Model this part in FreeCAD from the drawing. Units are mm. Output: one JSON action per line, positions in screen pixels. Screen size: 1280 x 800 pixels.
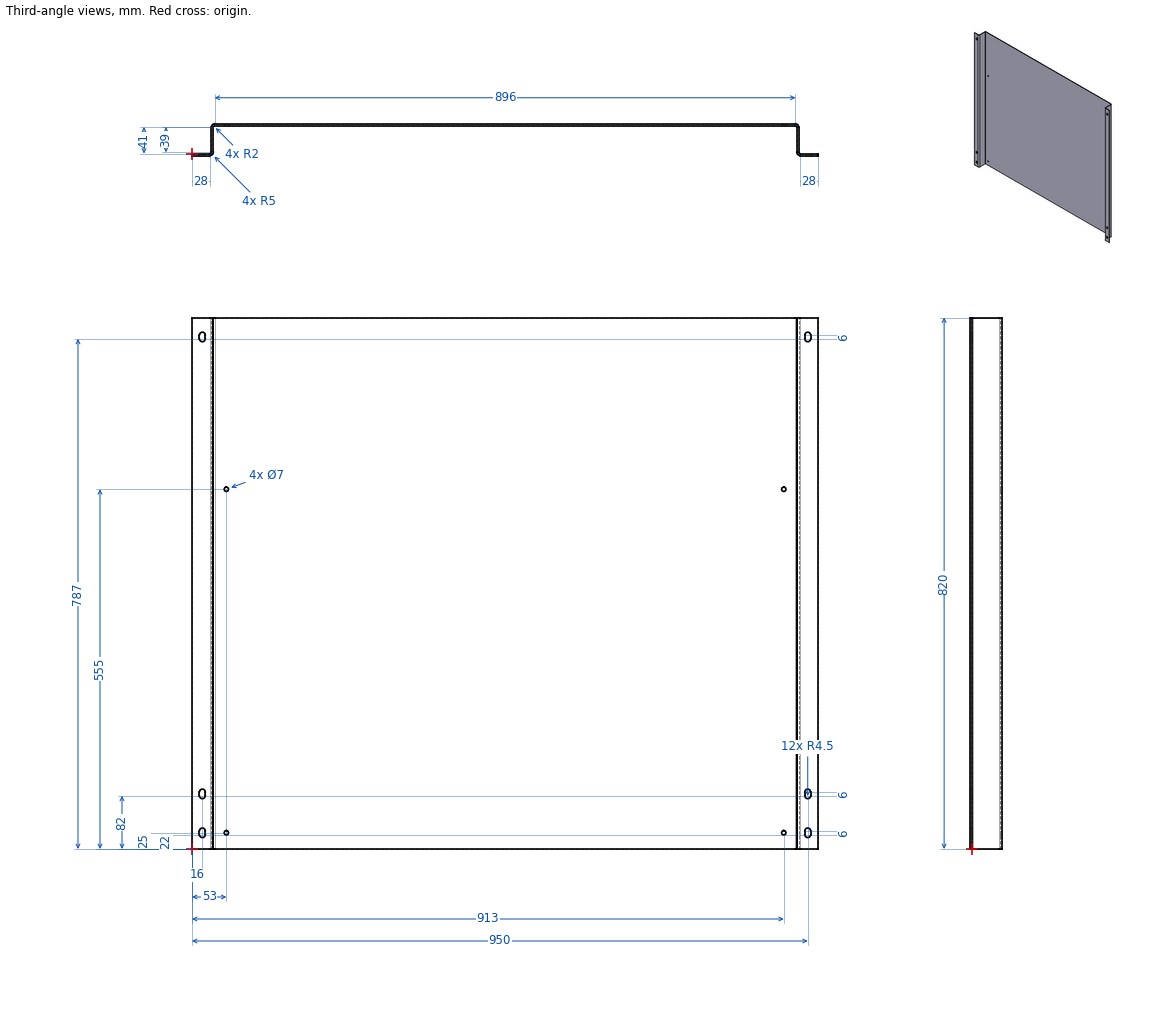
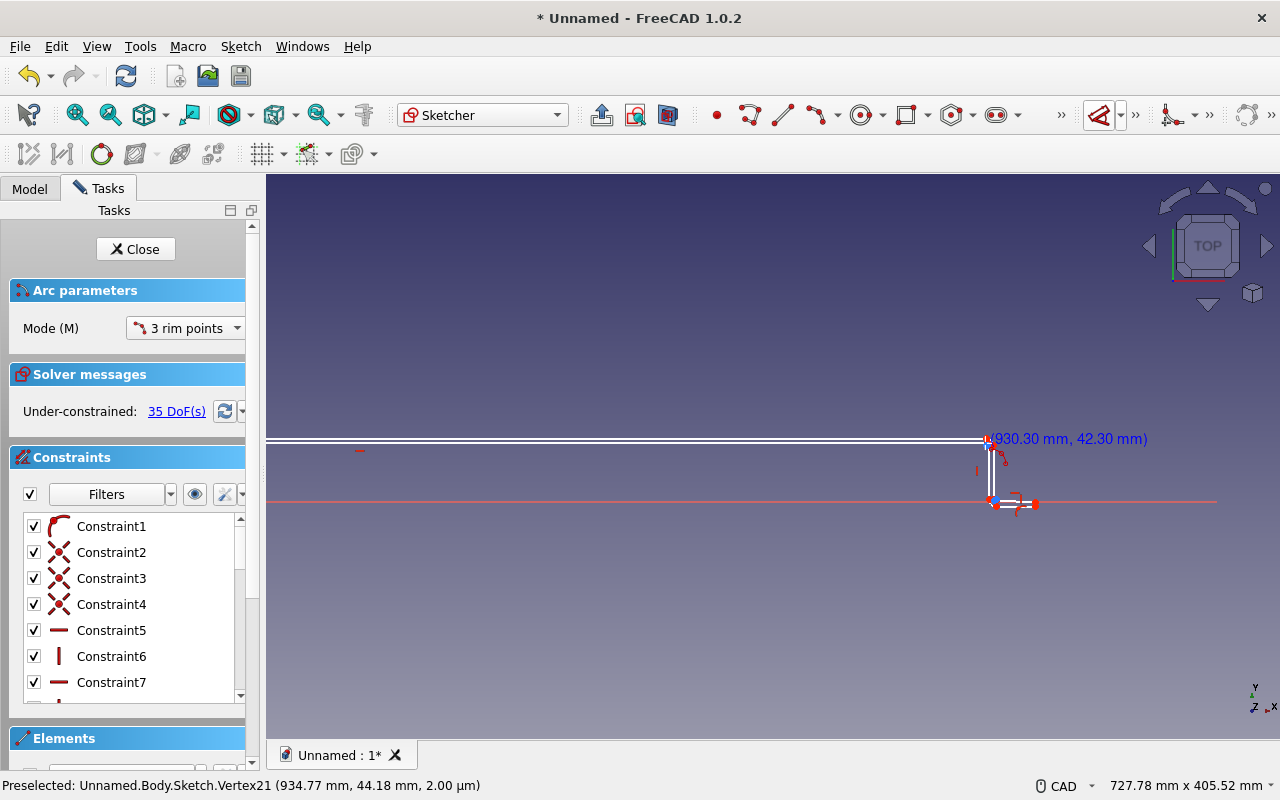
{"action": "scroll", "coordinate": [425, 441], "scroll_direction": "up", "scroll_amount": 11}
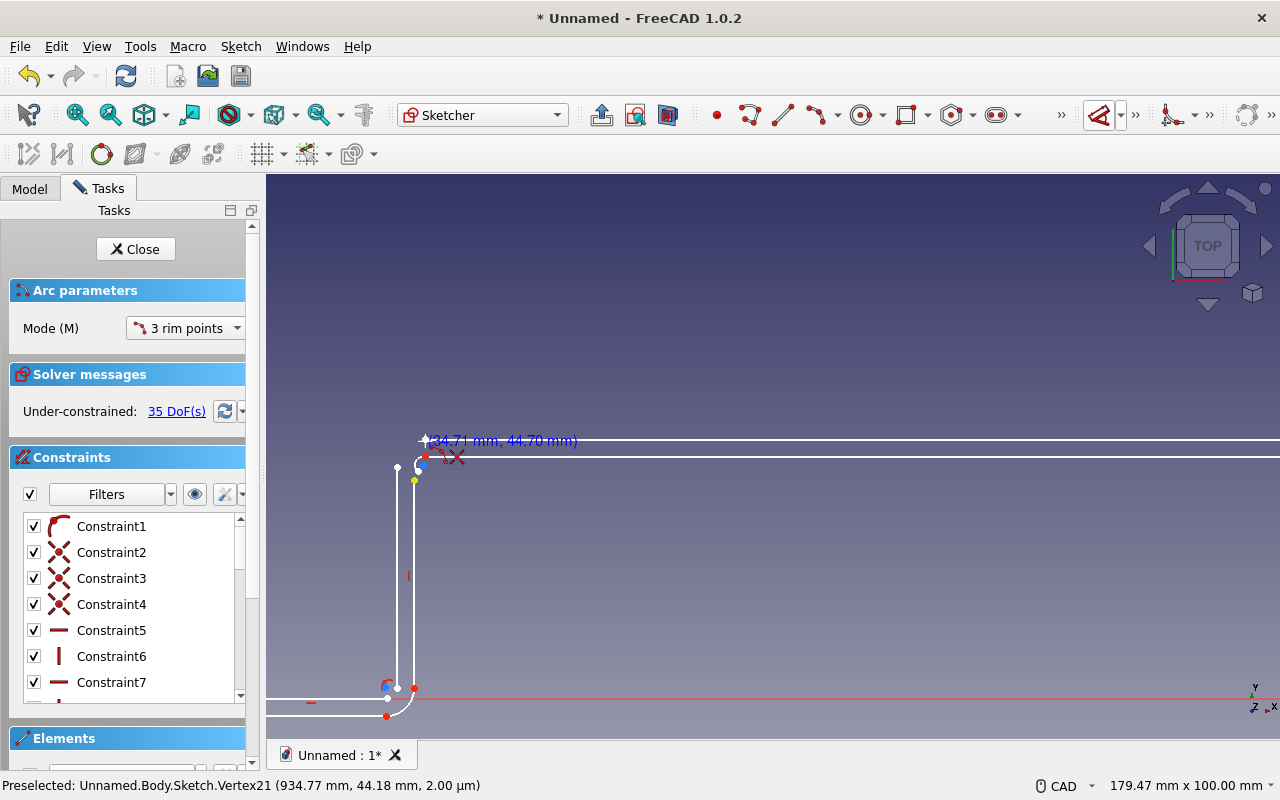
{"action": "left_click", "coordinate": [425, 440]}
{"action": "left_click", "coordinate": [397, 468]}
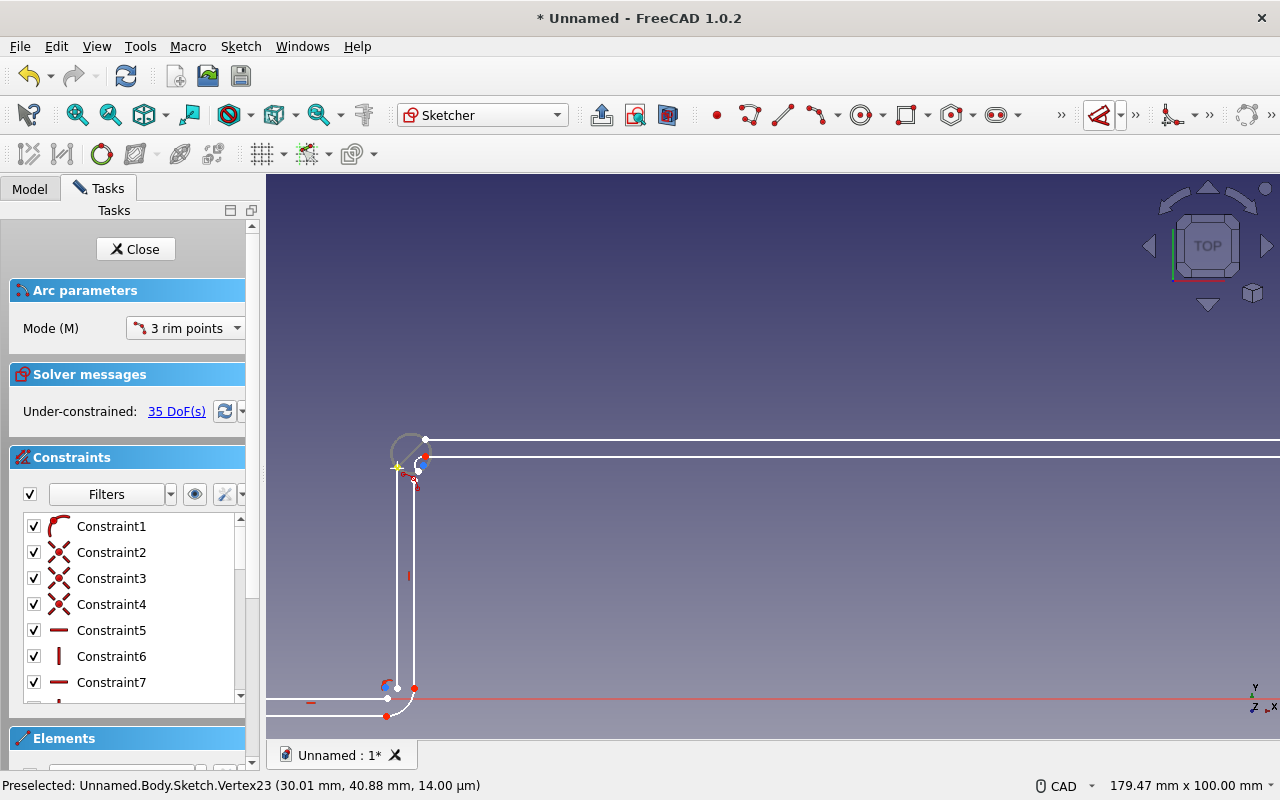
{"action": "scroll", "coordinate": [405, 447], "scroll_direction": "up", "scroll_amount": 4}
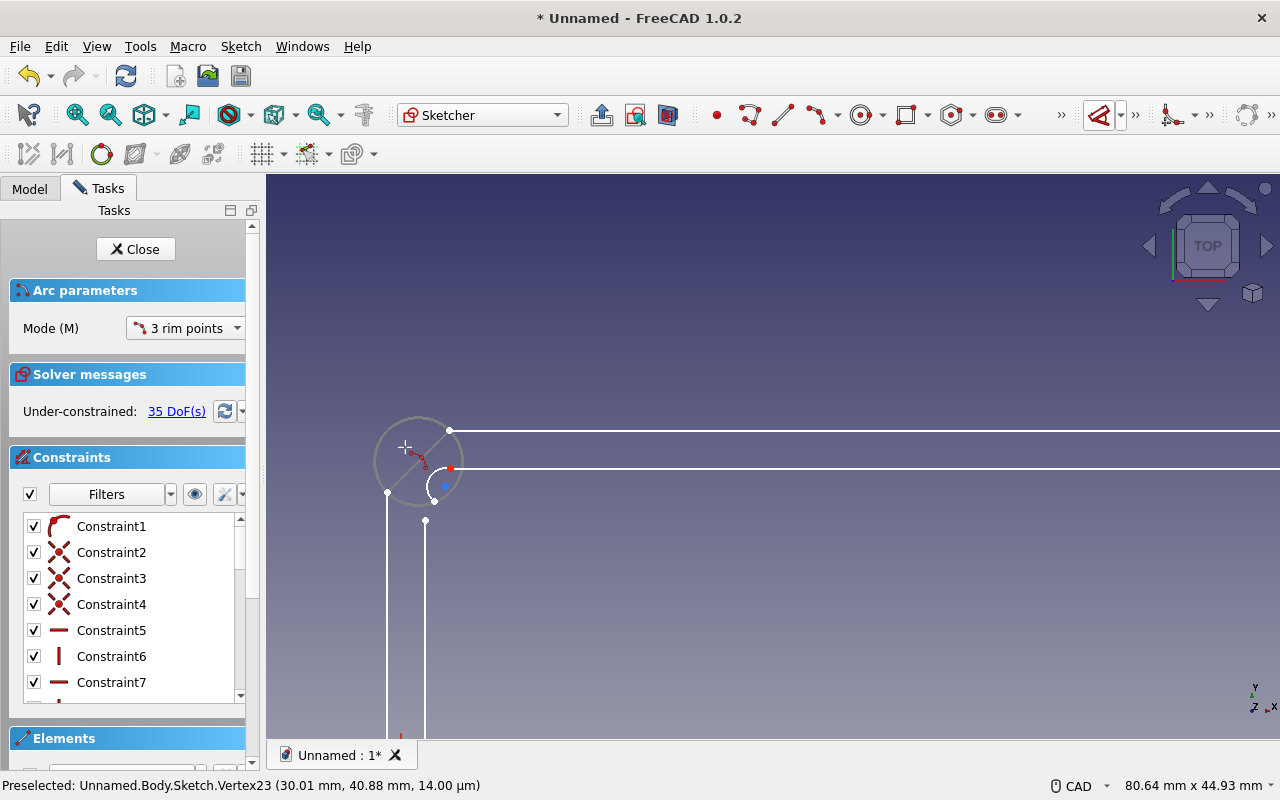
{"action": "left_click", "coordinate": [406, 447]}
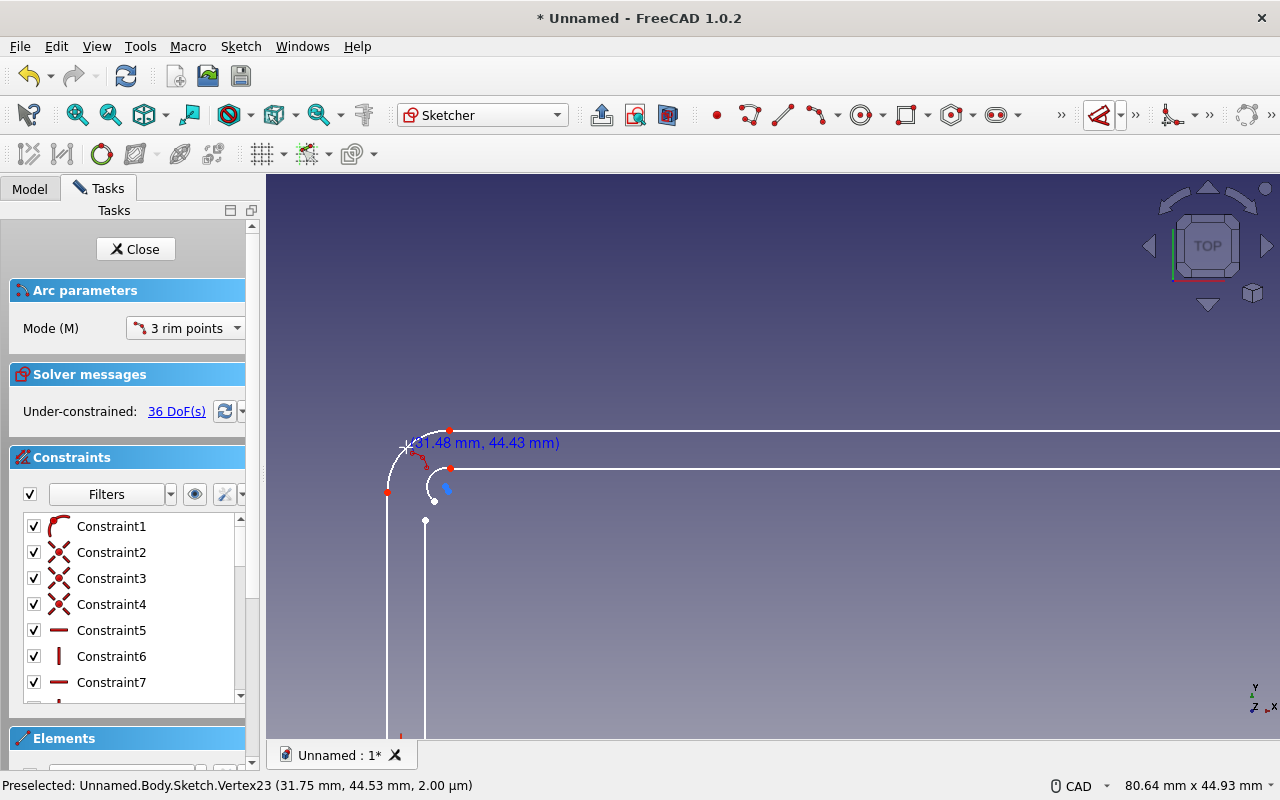
{"action": "scroll", "coordinate": [423, 442], "scroll_direction": "down", "scroll_amount": 15}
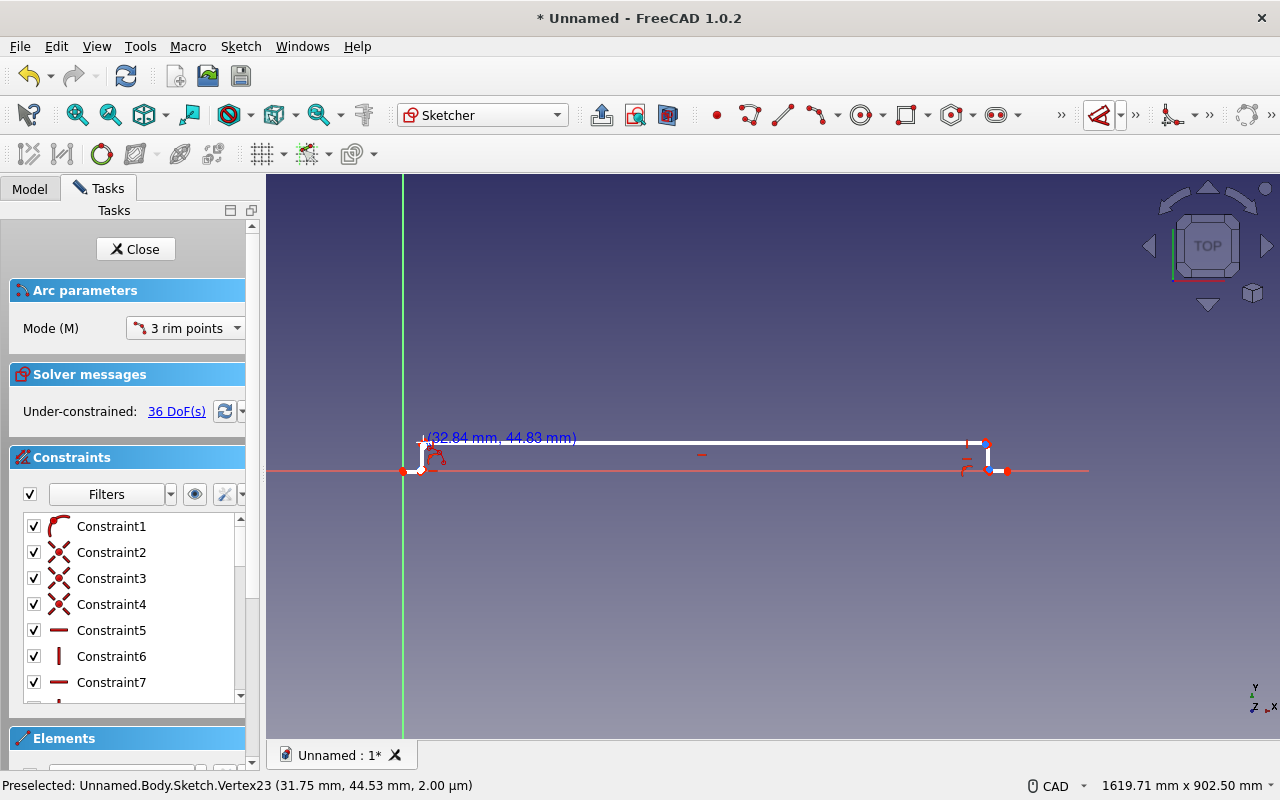
{"action": "scroll", "coordinate": [421, 469], "scroll_direction": "up", "scroll_amount": 13}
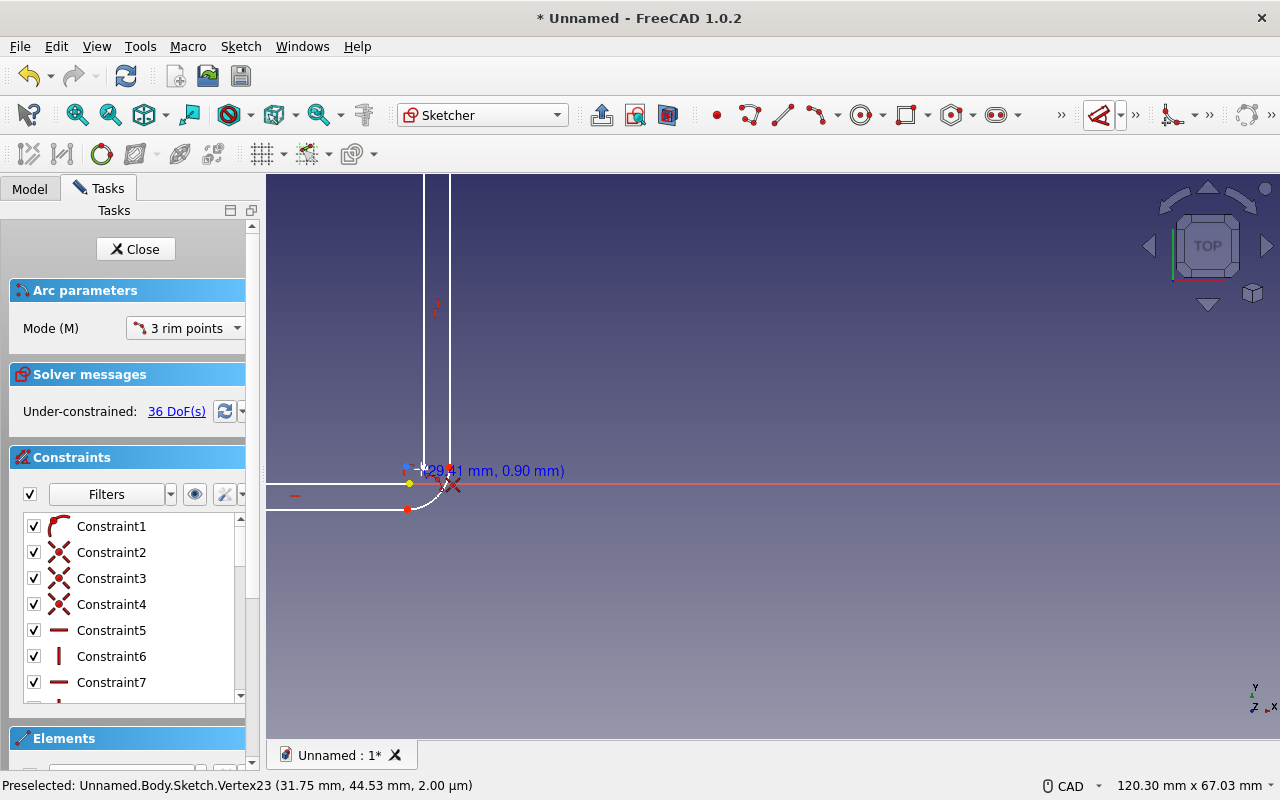
{"action": "left_click", "coordinate": [424, 468]}
{"action": "left_click", "coordinate": [410, 484]}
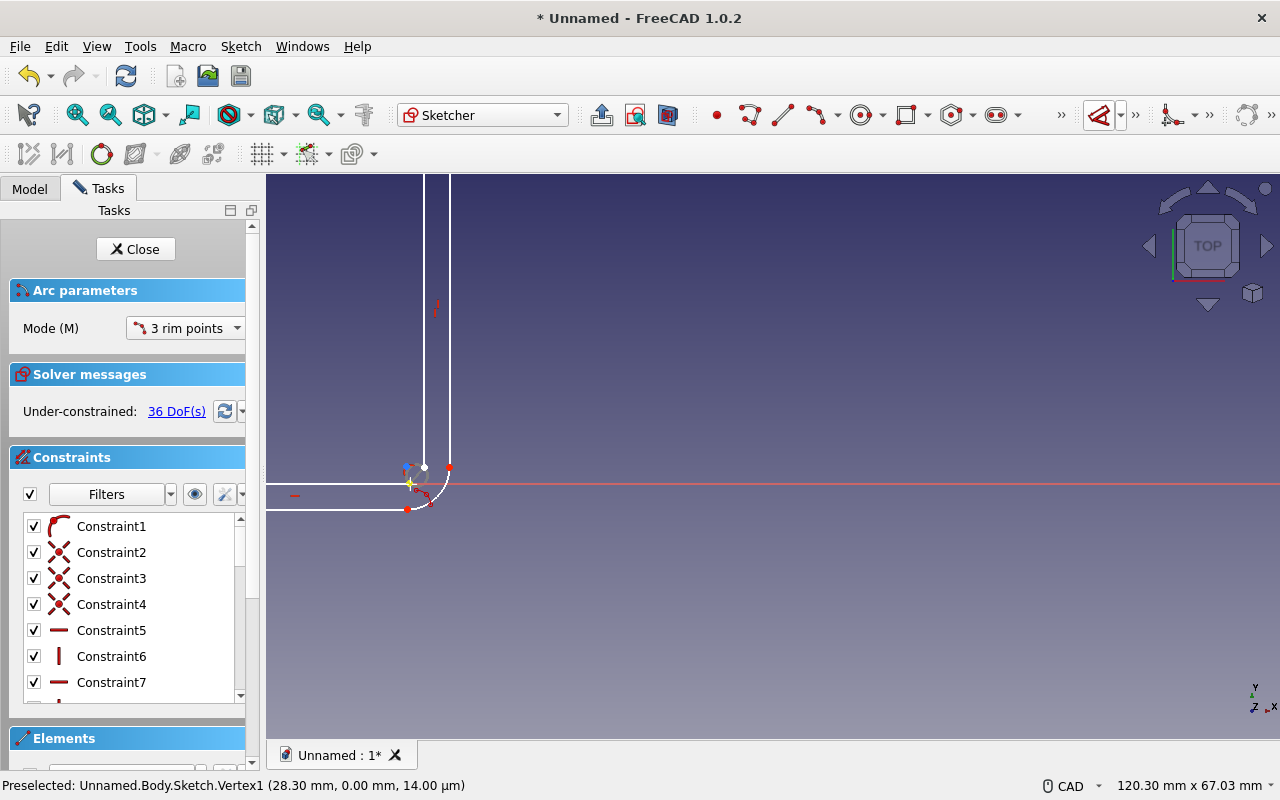
{"action": "scroll", "coordinate": [419, 479], "scroll_direction": "up", "scroll_amount": 6}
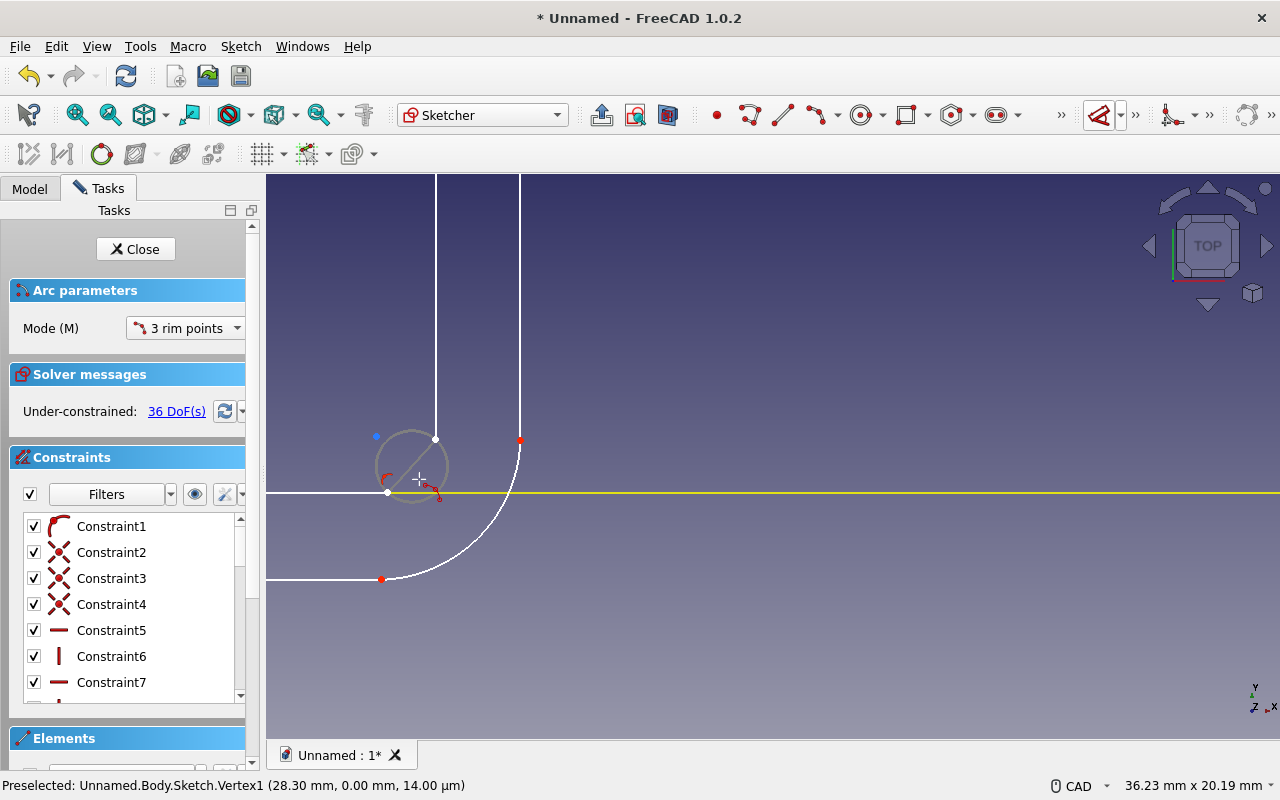
{"action": "left_click", "coordinate": [419, 477]}
{"action": "key", "text": "Escape"}